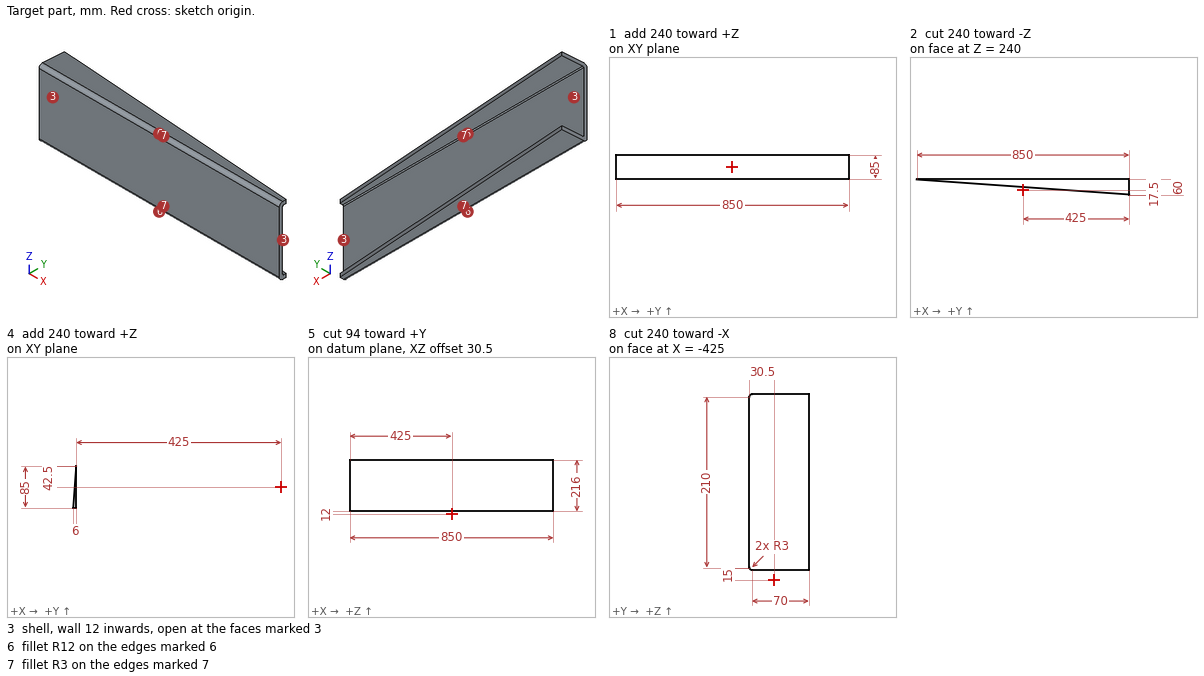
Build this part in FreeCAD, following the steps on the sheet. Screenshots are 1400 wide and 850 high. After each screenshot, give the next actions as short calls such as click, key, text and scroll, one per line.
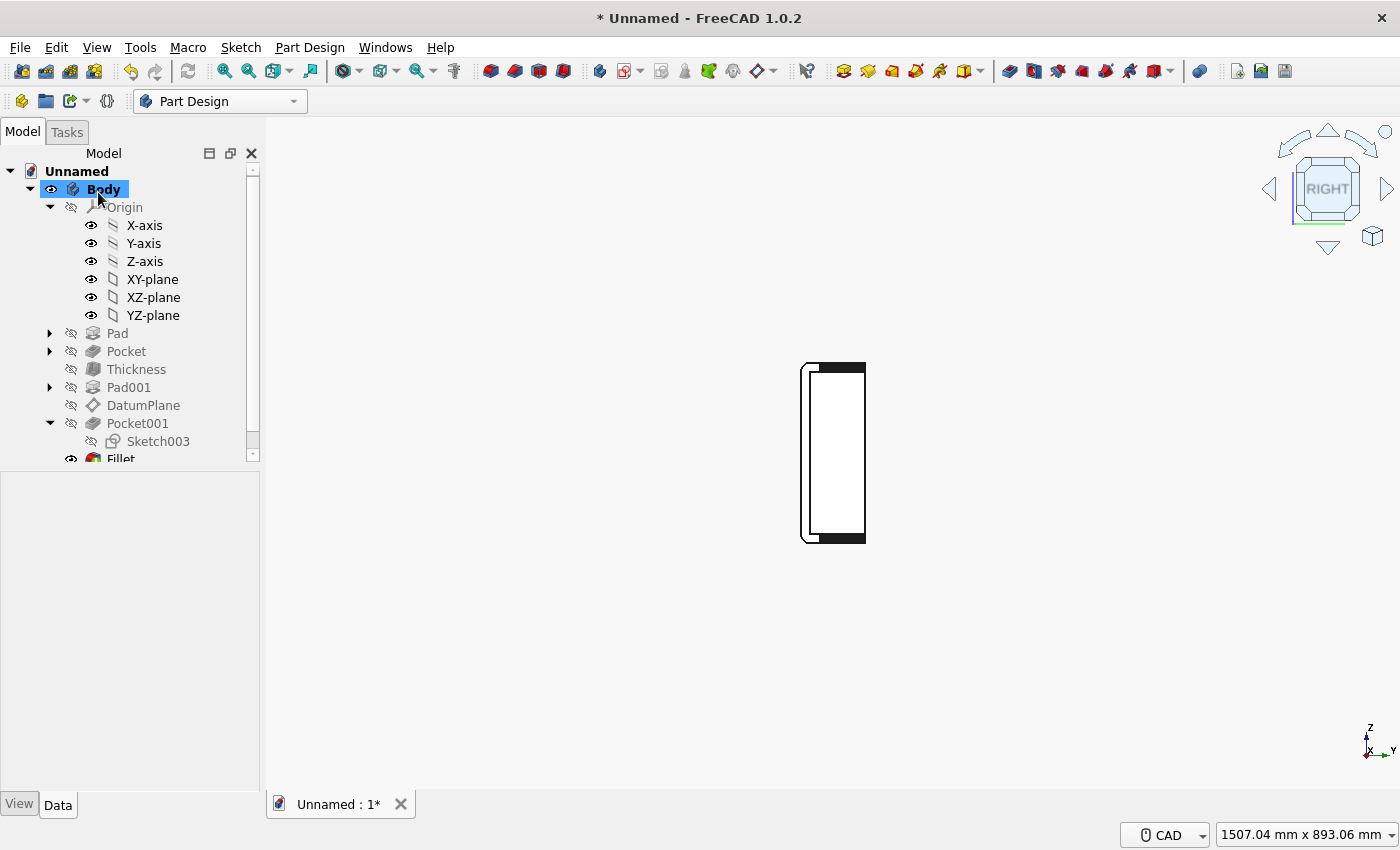
key(5)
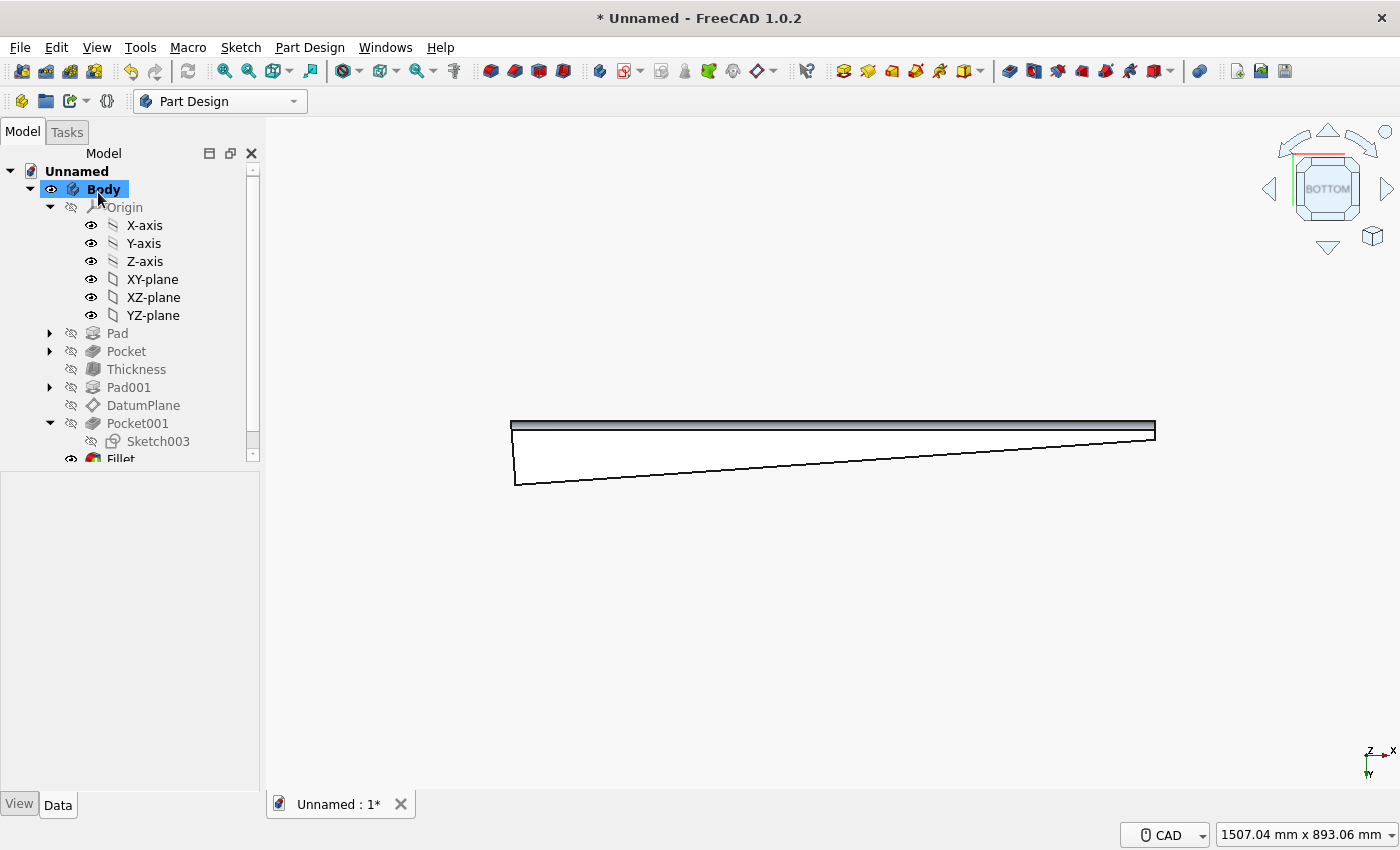
key(4)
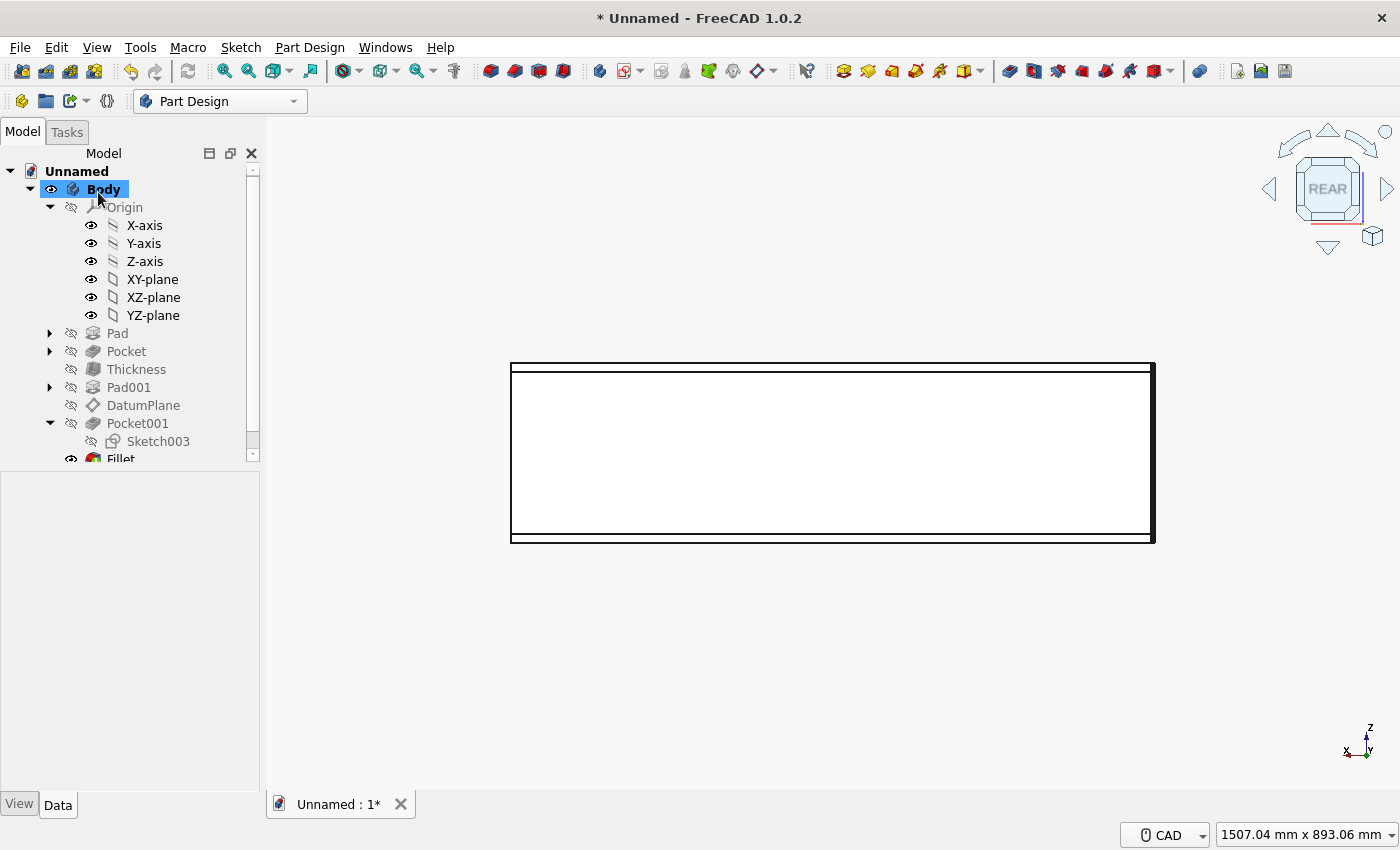
key(6)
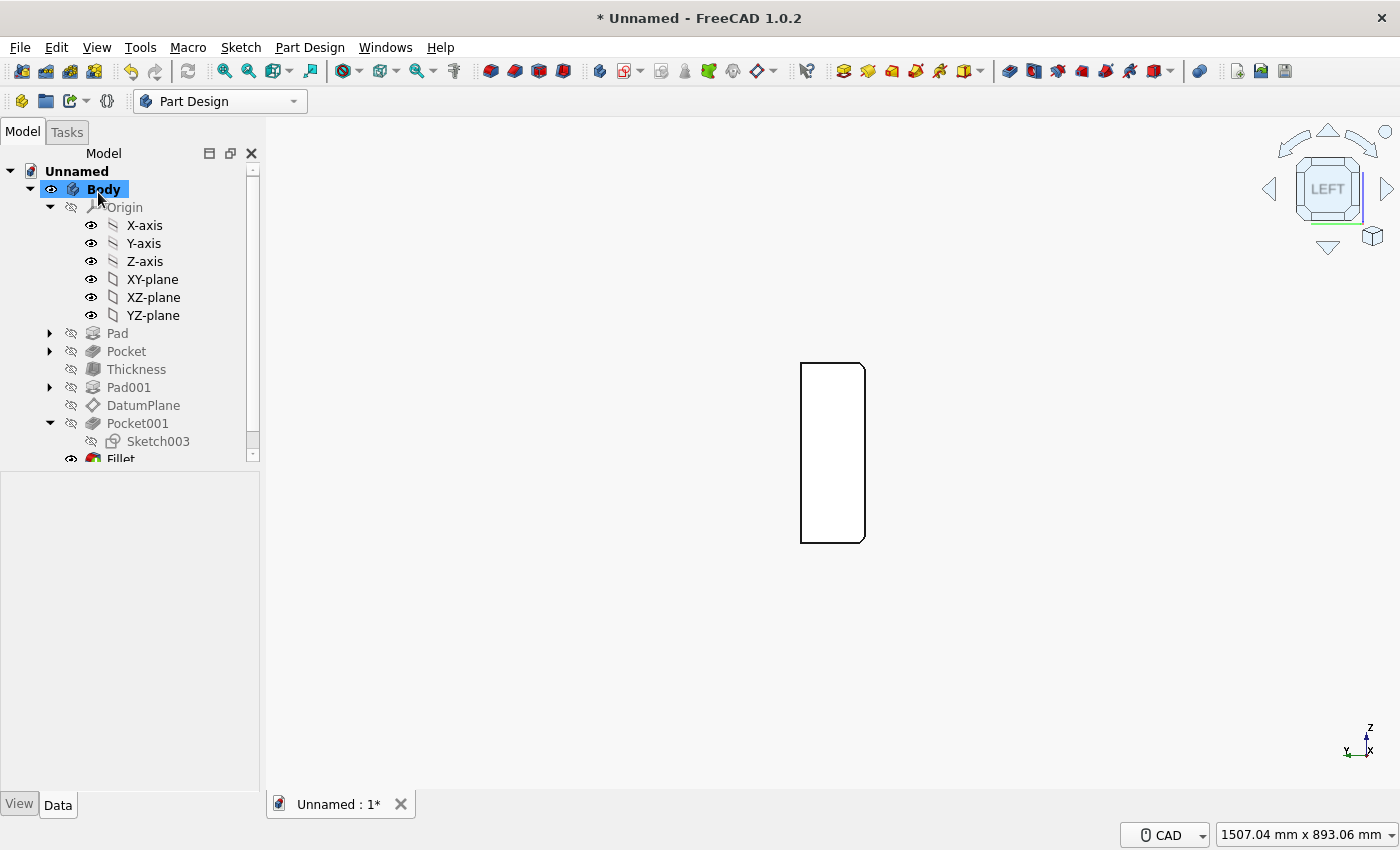
click(226, 72)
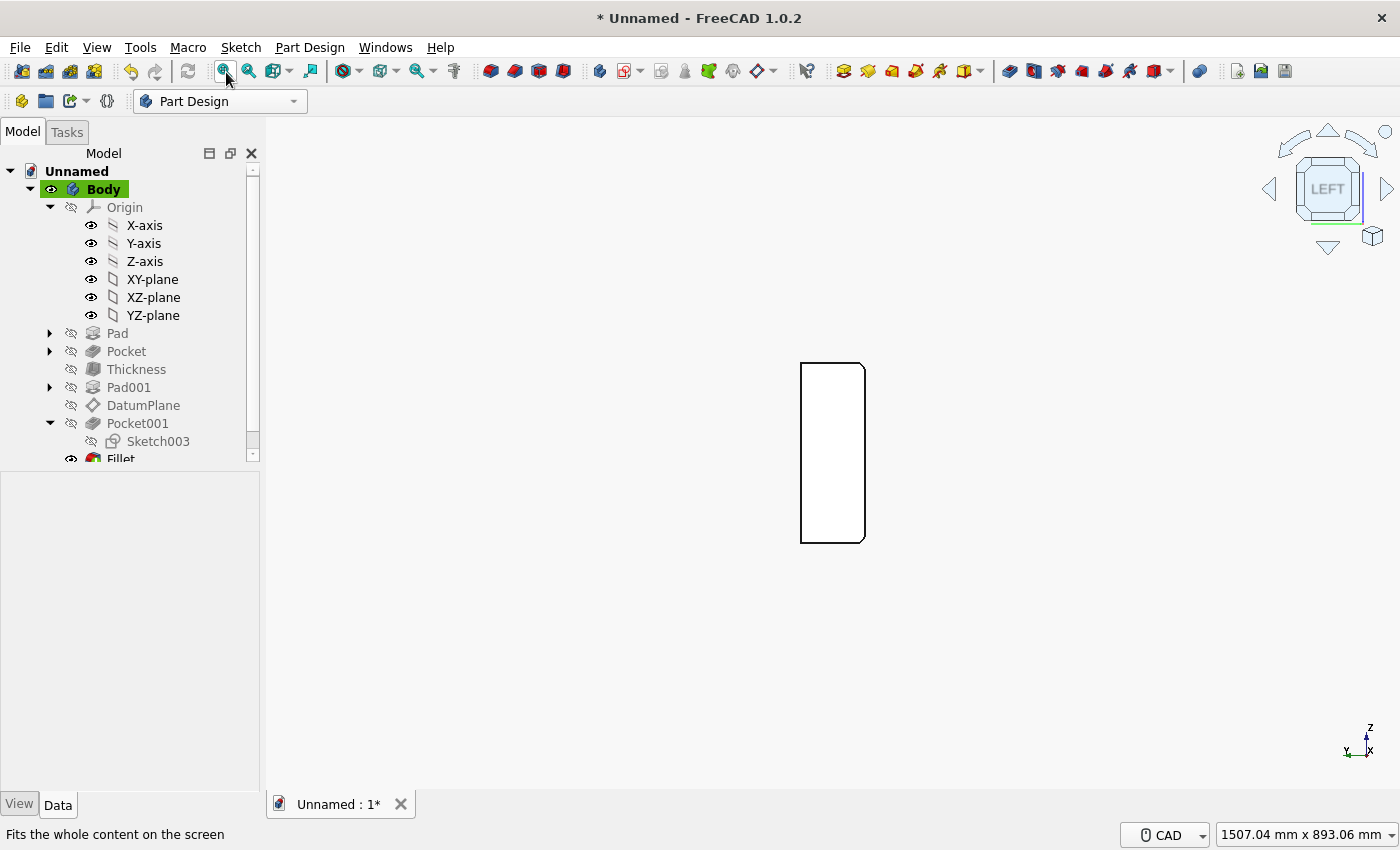
key(v)
key(3)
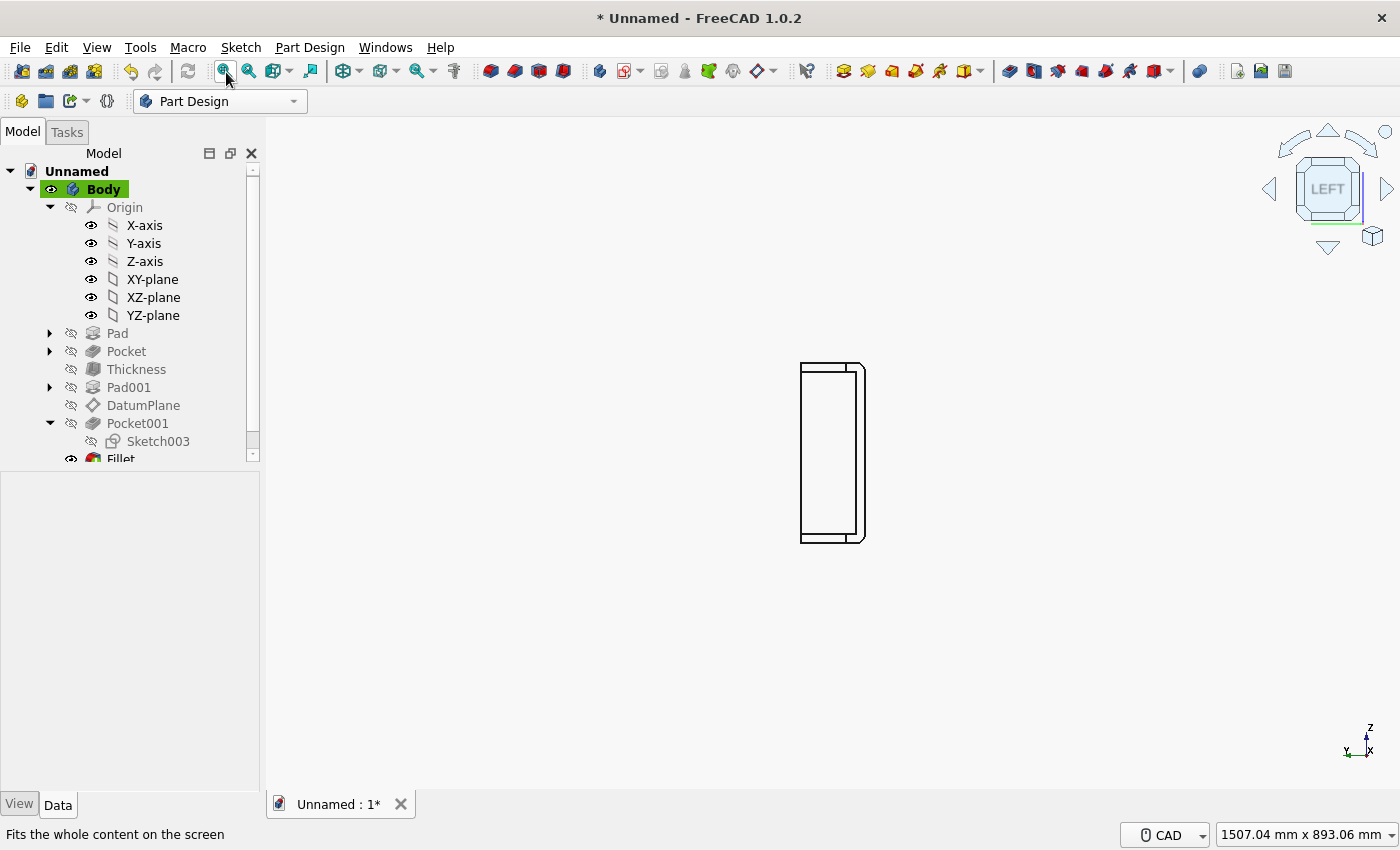
key(0)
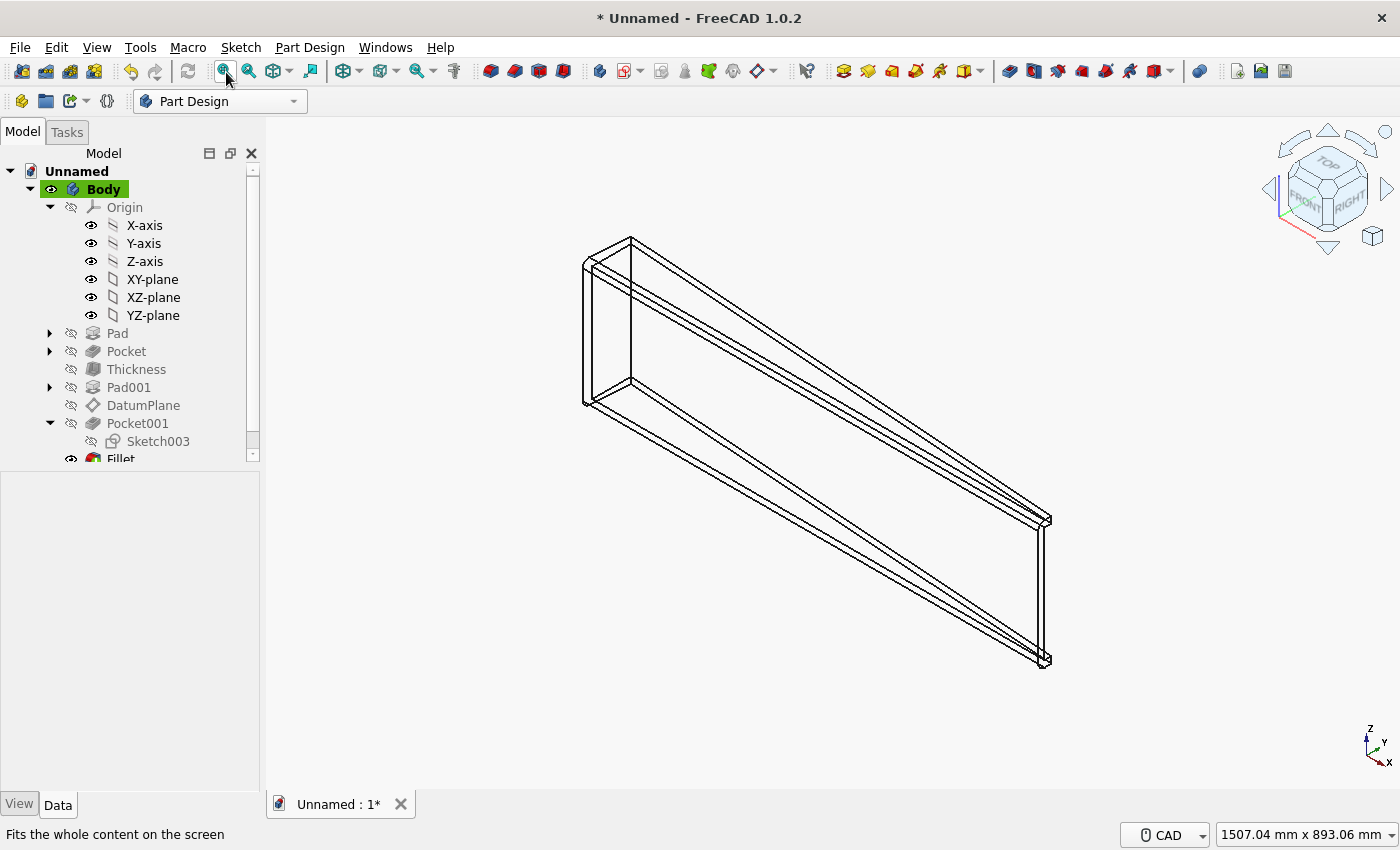
click(864, 555)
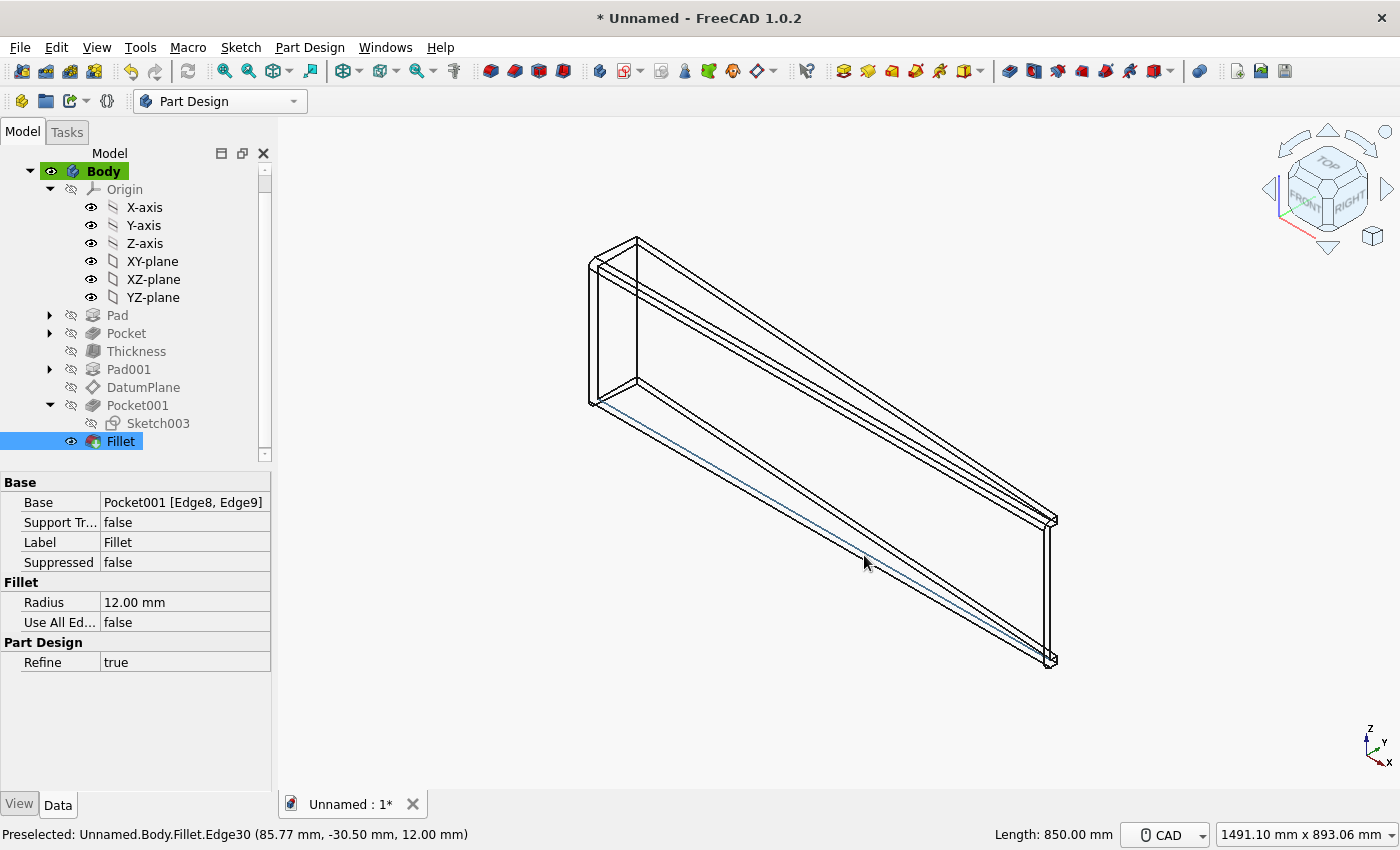
click(653, 297, ctrl)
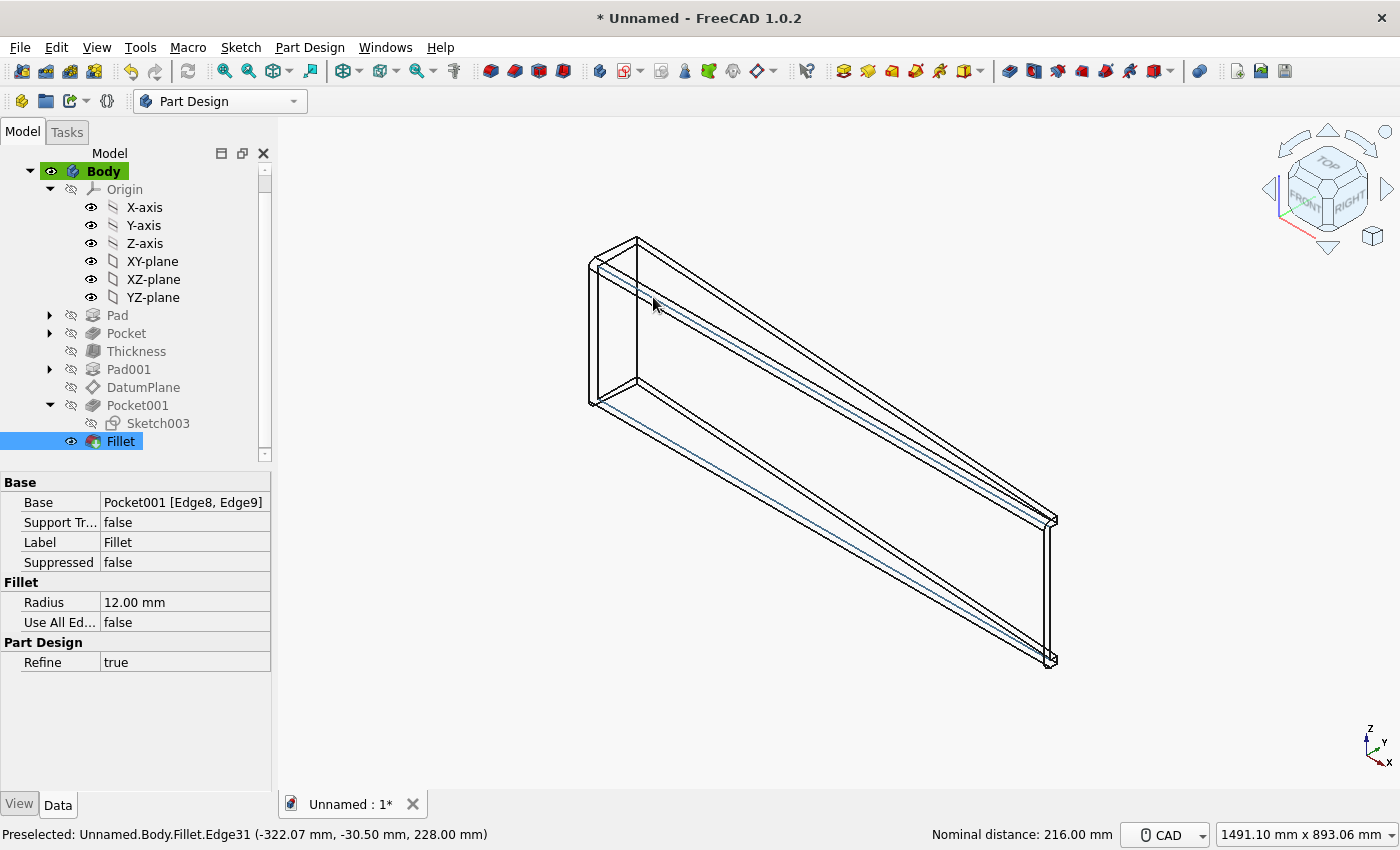
key(v)
key(1)